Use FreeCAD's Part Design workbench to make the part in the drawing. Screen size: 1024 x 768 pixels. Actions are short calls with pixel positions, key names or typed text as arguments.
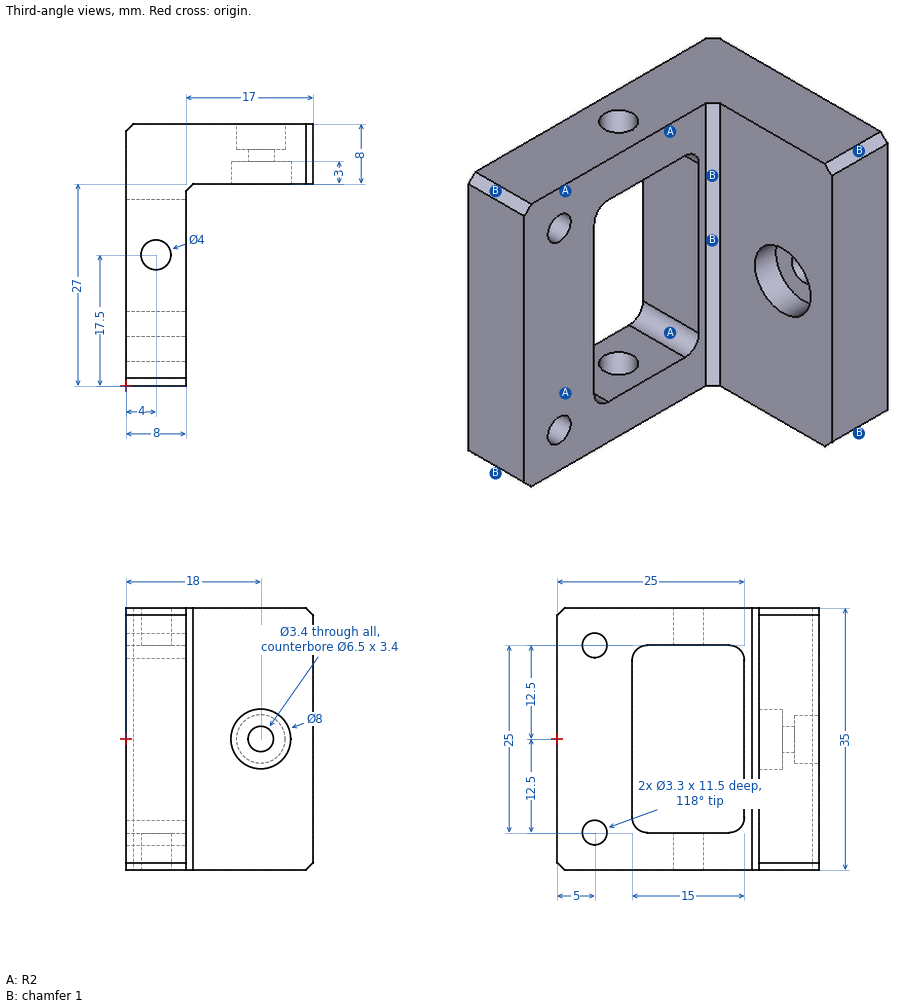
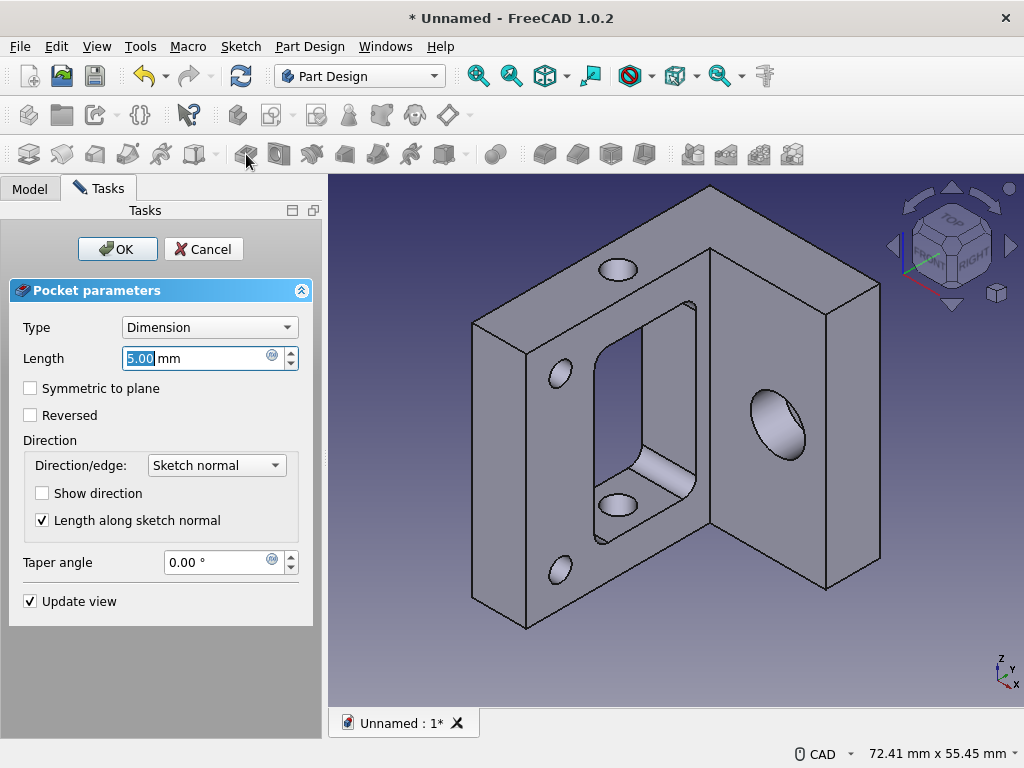
text(3)
key(Tab)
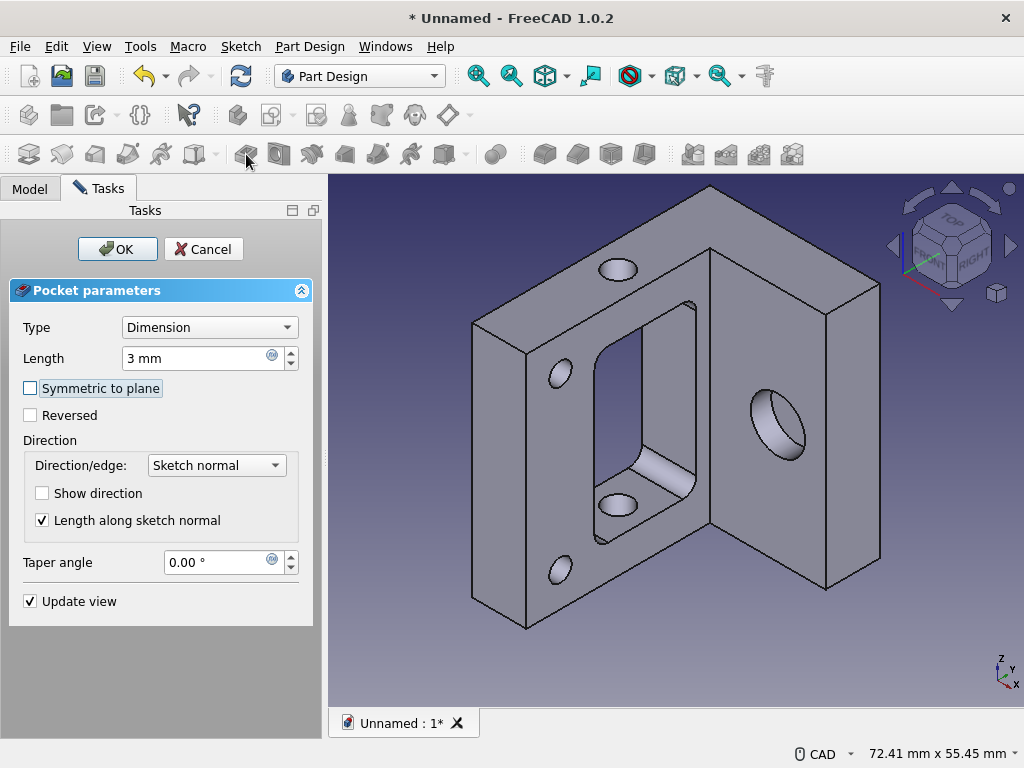
click(118, 249)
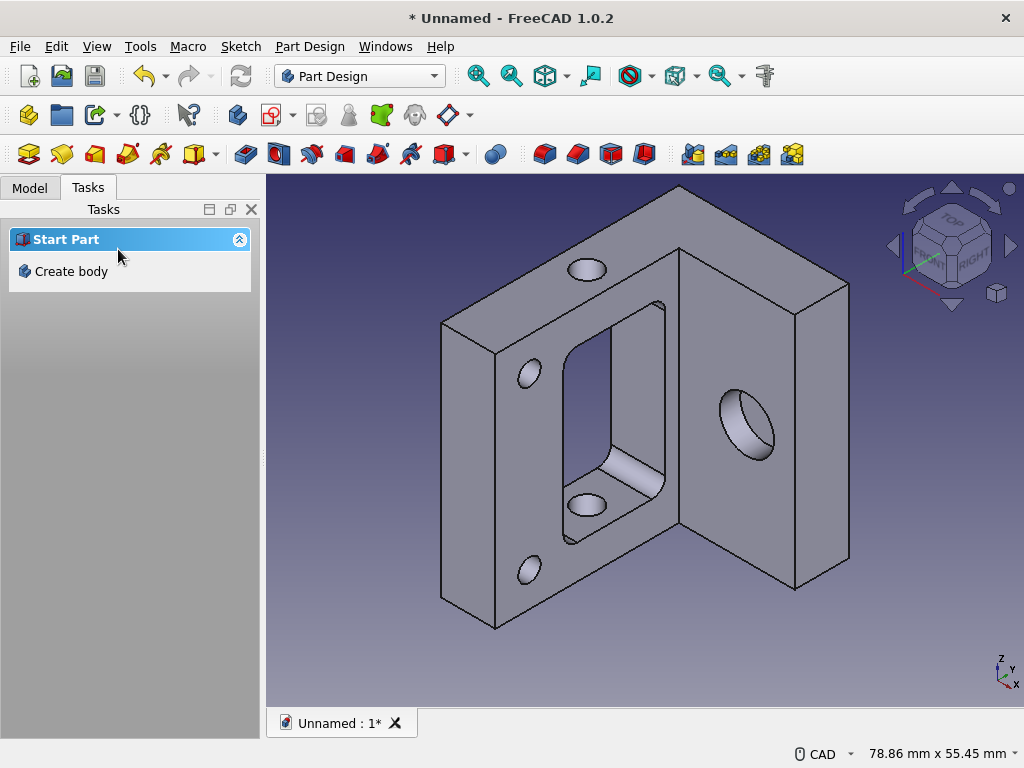
click(822, 298)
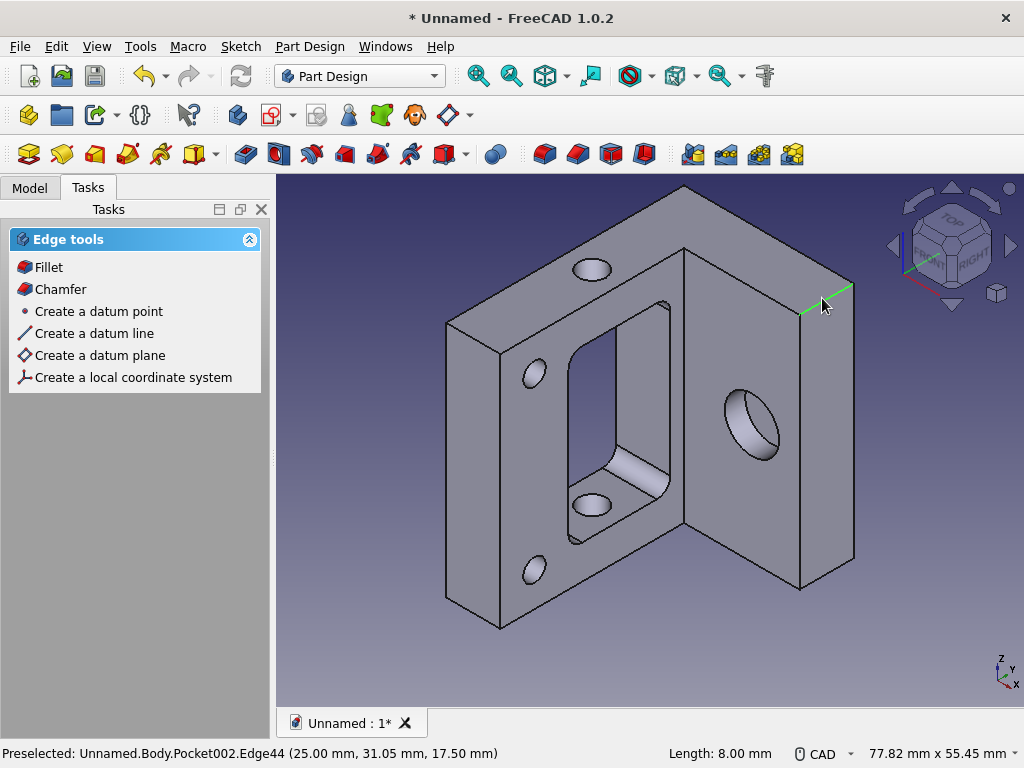
click(473, 337, ctrl)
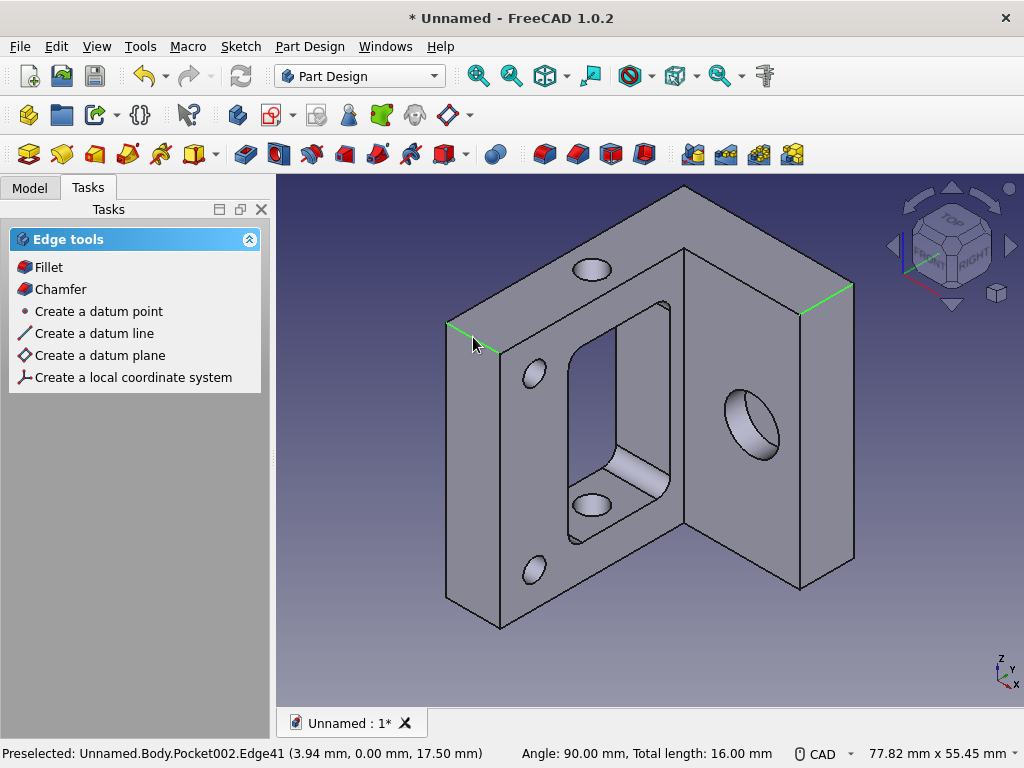
key(2)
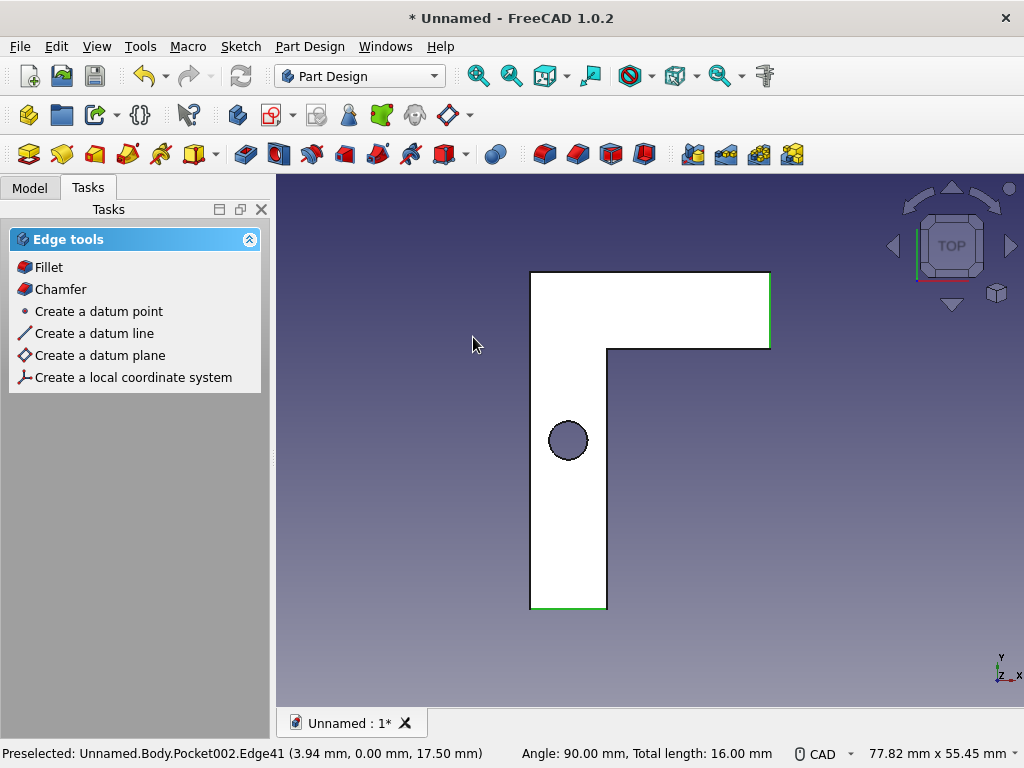
key(0)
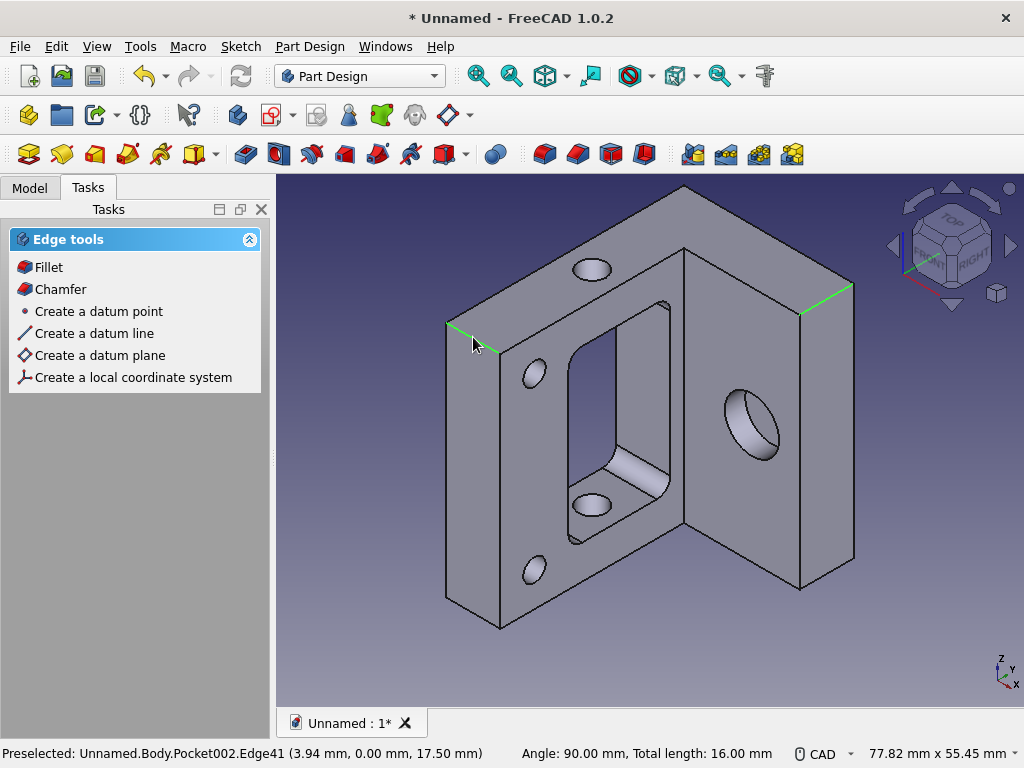
key(1)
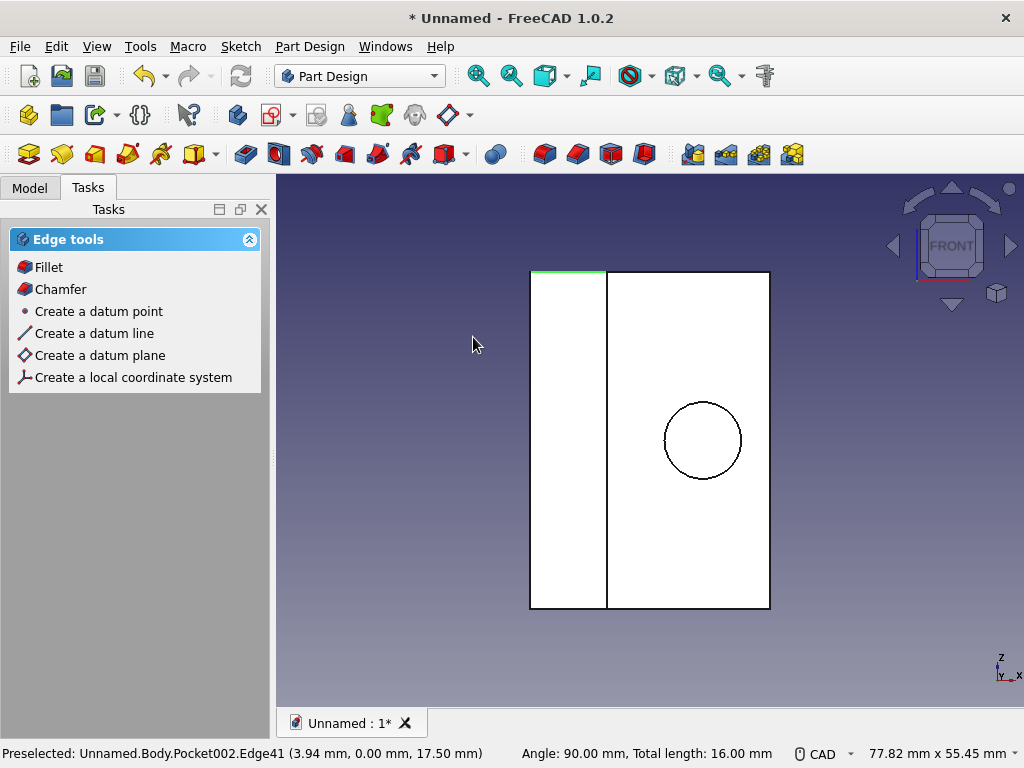
click(568, 608, ctrl)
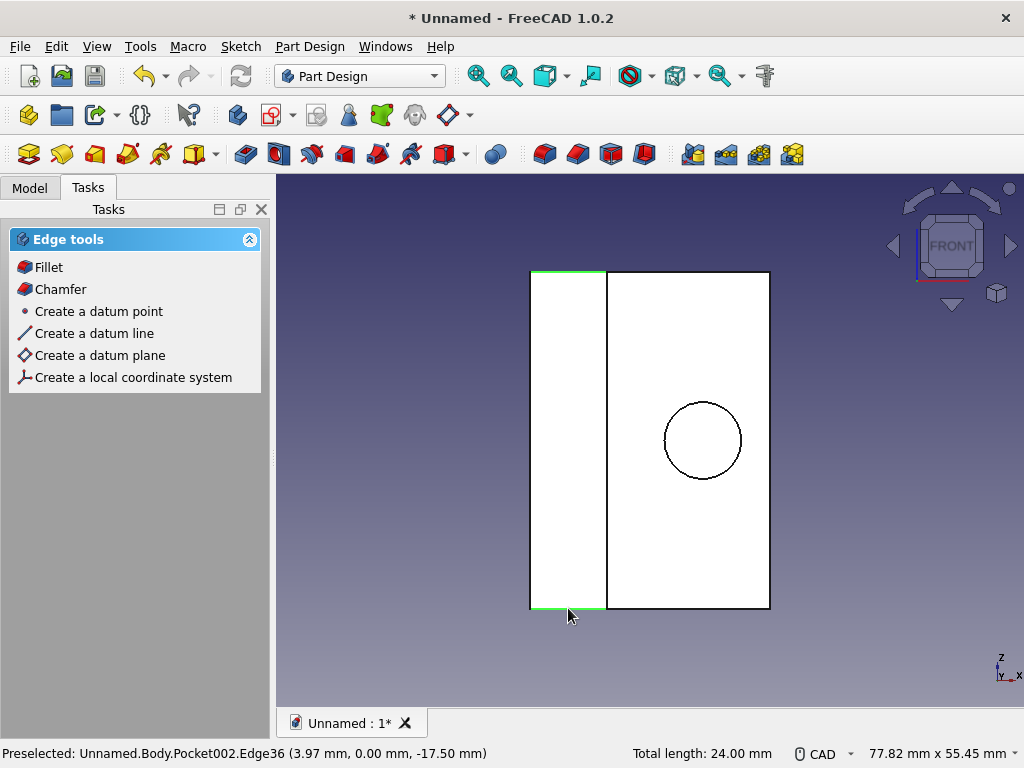
key(3)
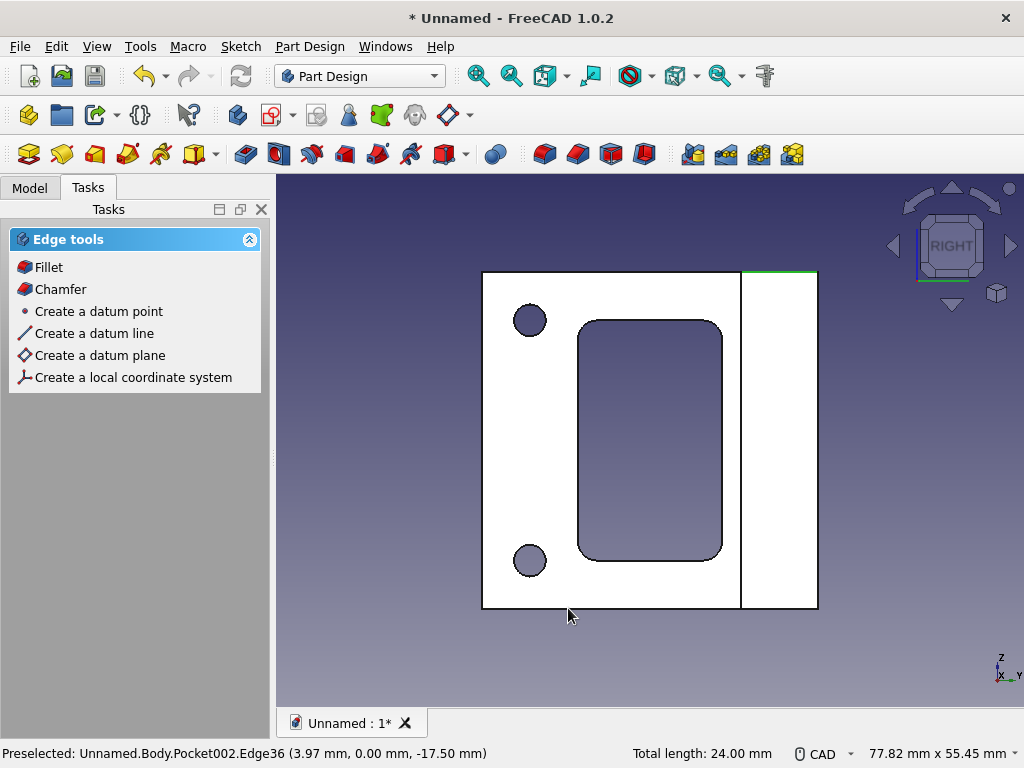
click(780, 608, ctrl)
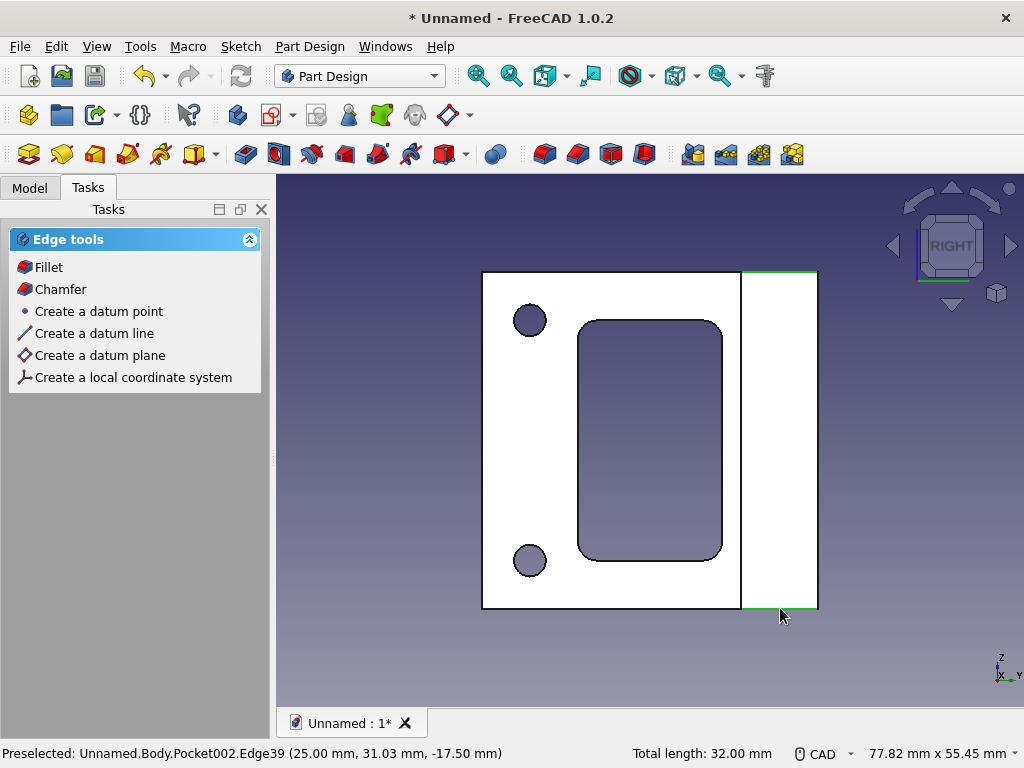
key(5)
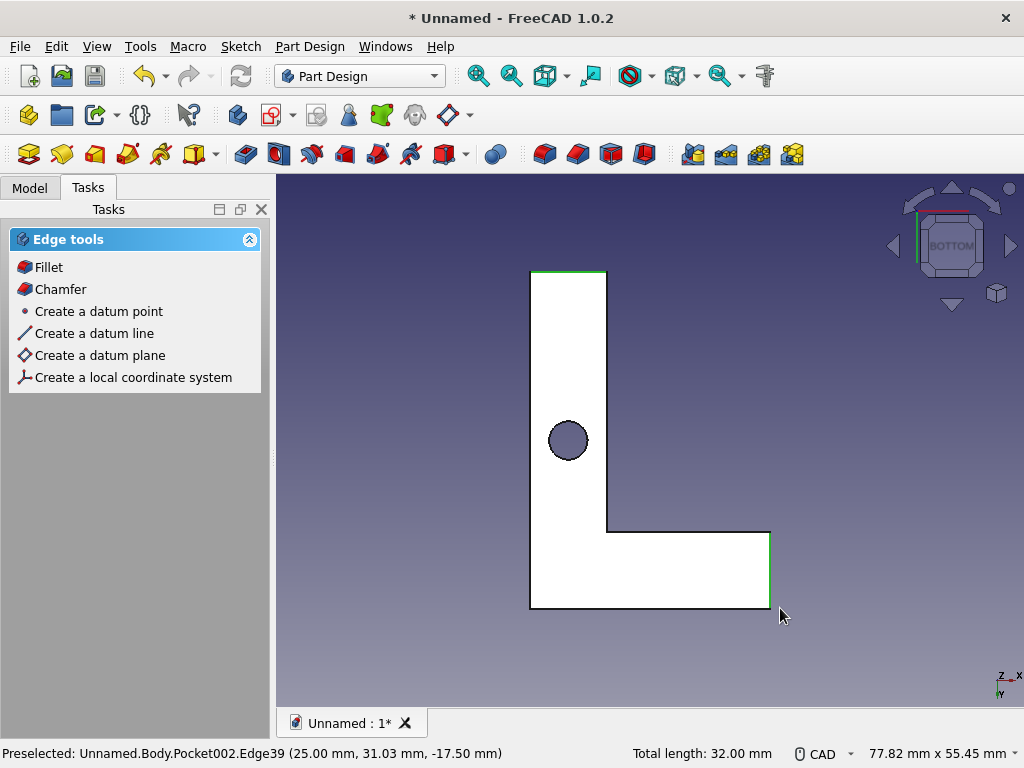
key(4)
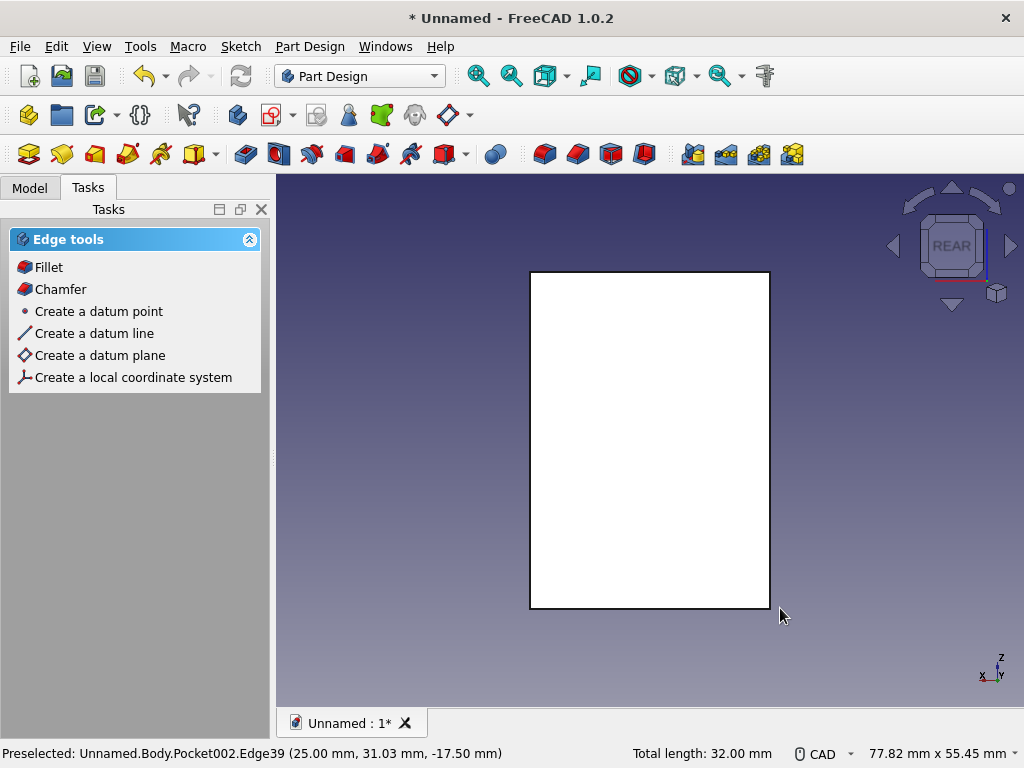
click(770, 439, ctrl)